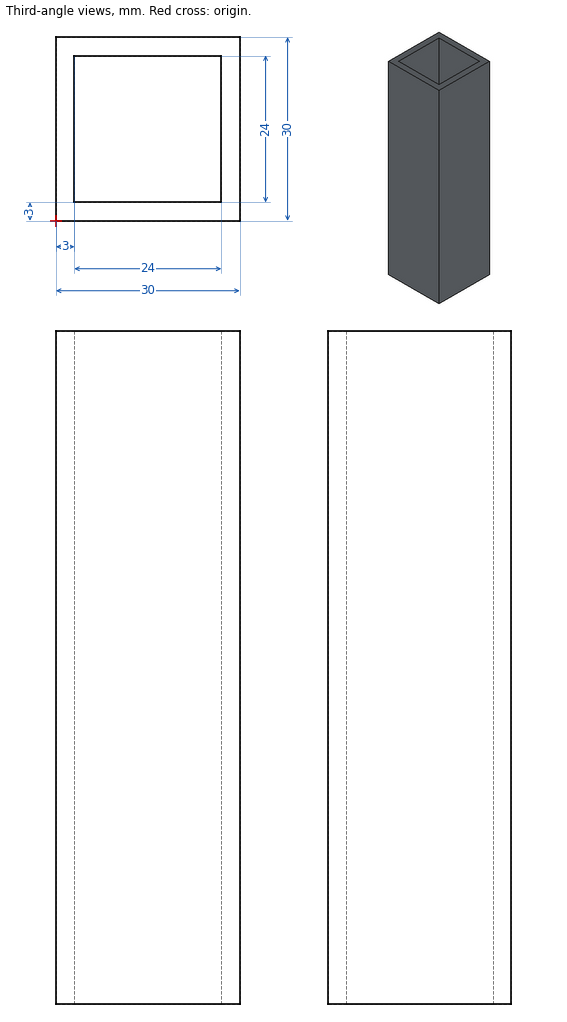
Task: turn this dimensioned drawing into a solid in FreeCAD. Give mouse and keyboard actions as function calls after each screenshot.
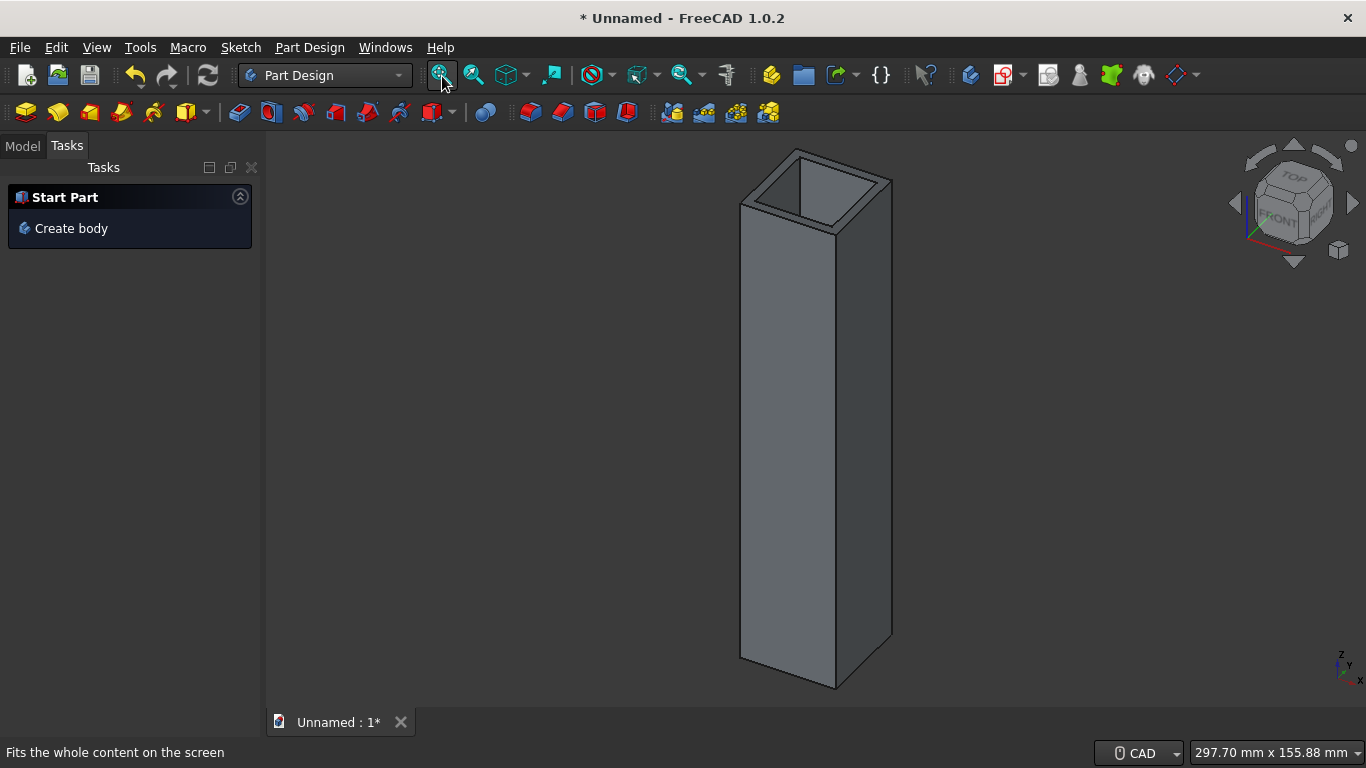
key(5)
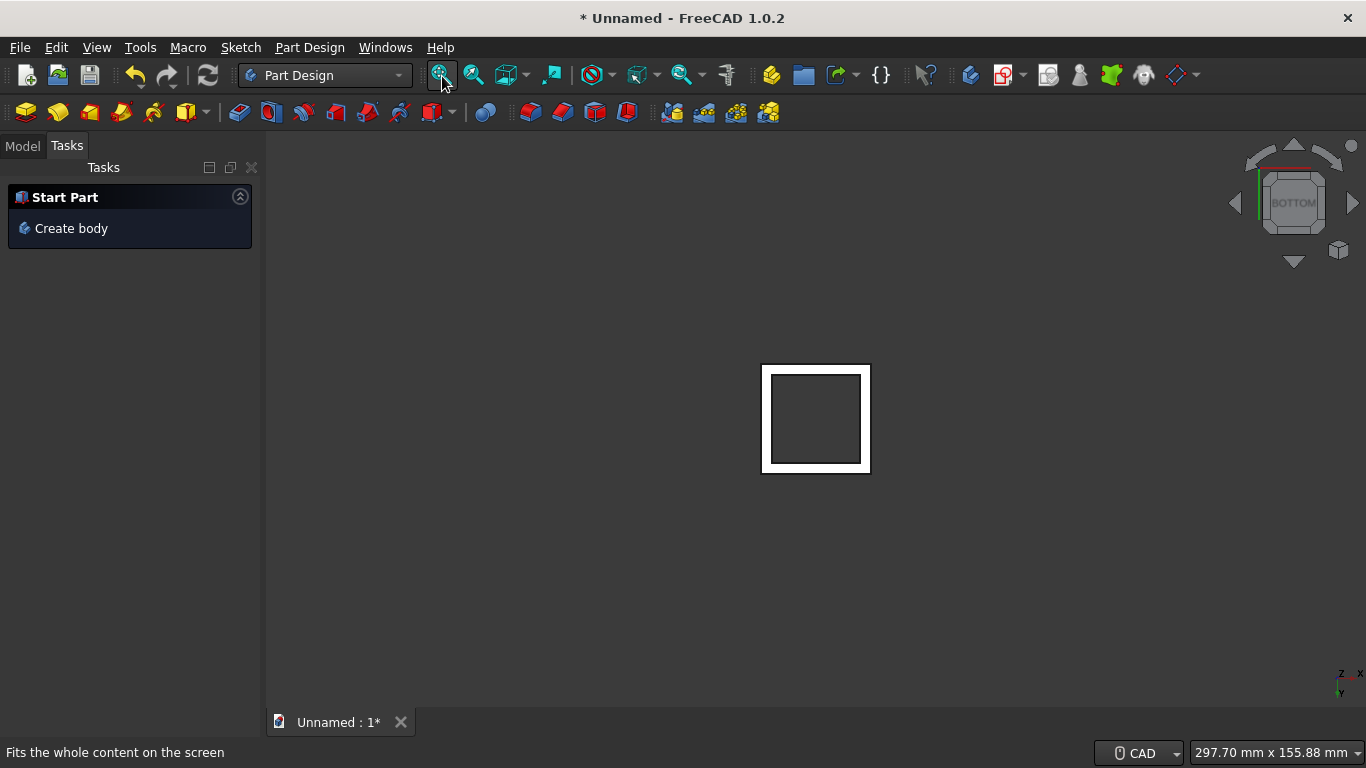
click(442, 76)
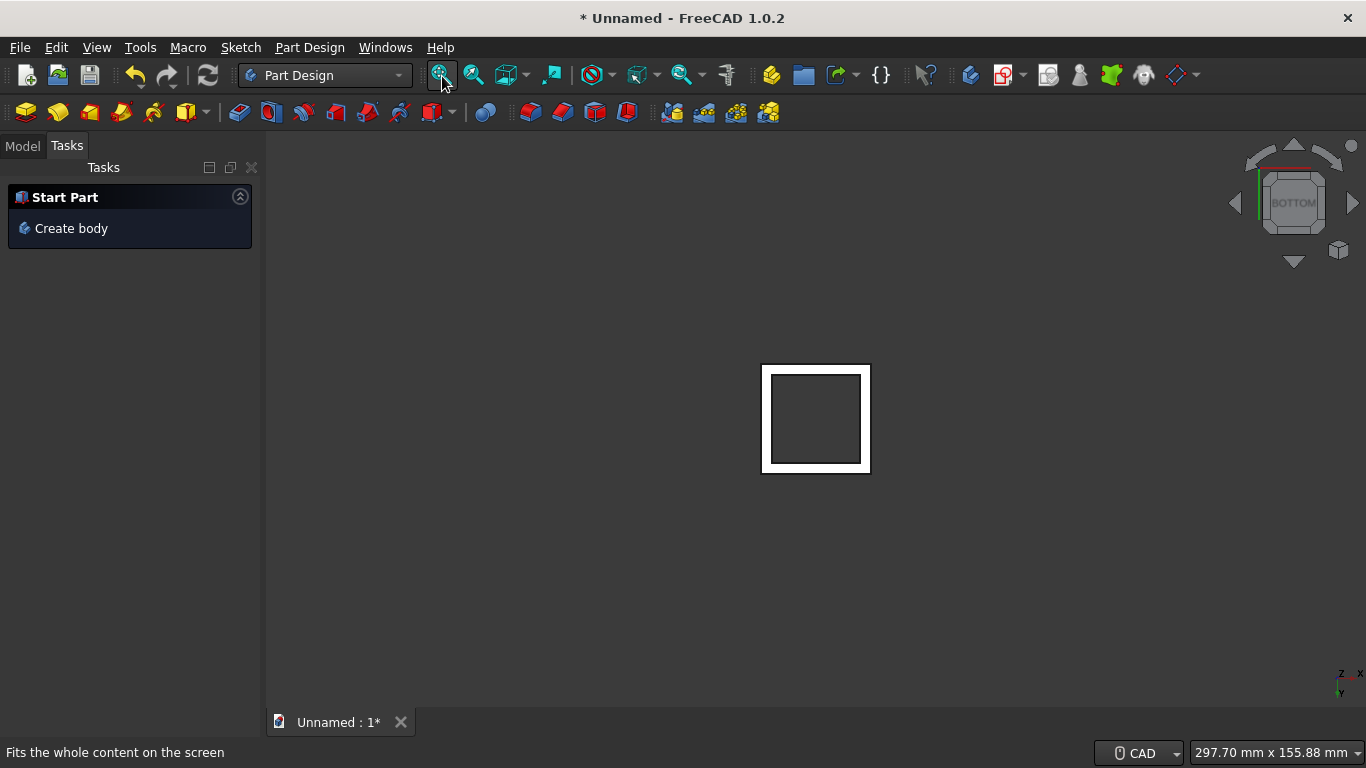
scroll(864, 466, up, 5)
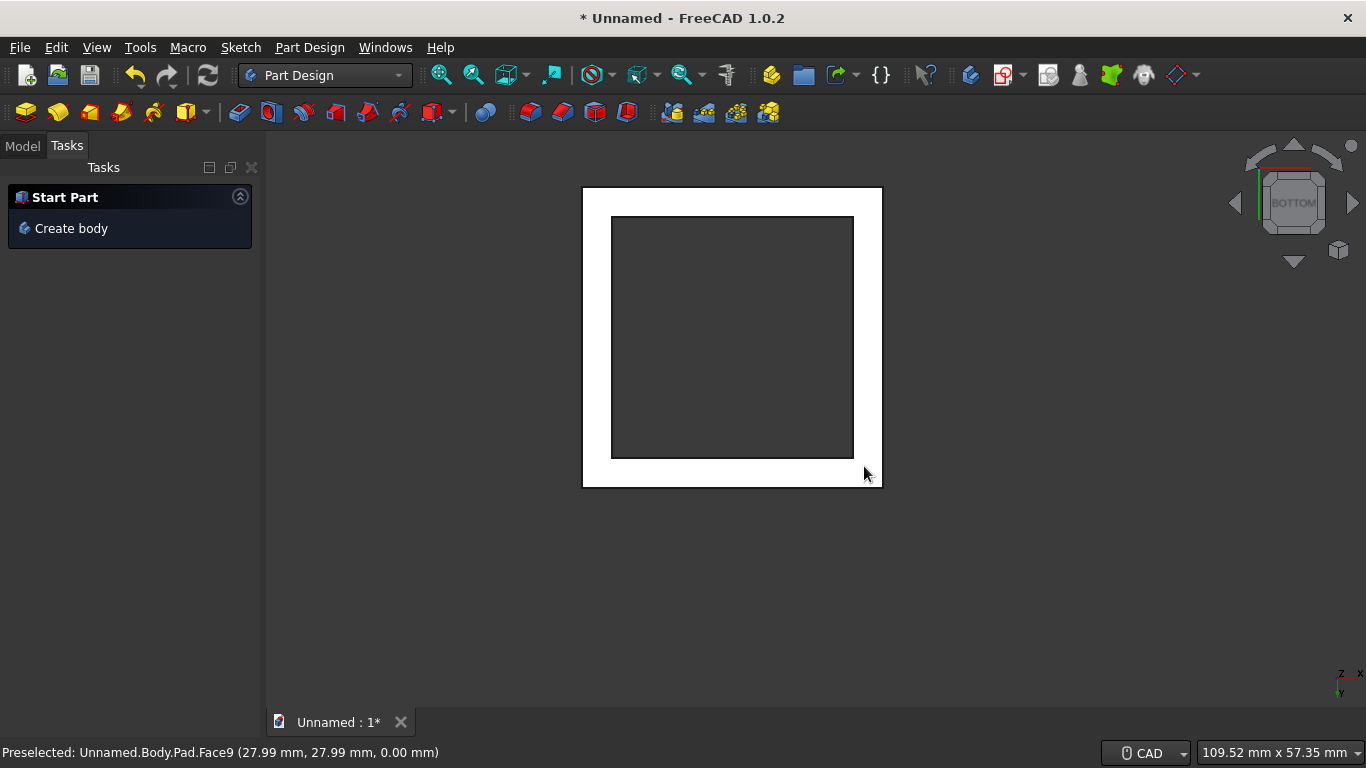
click(862, 465)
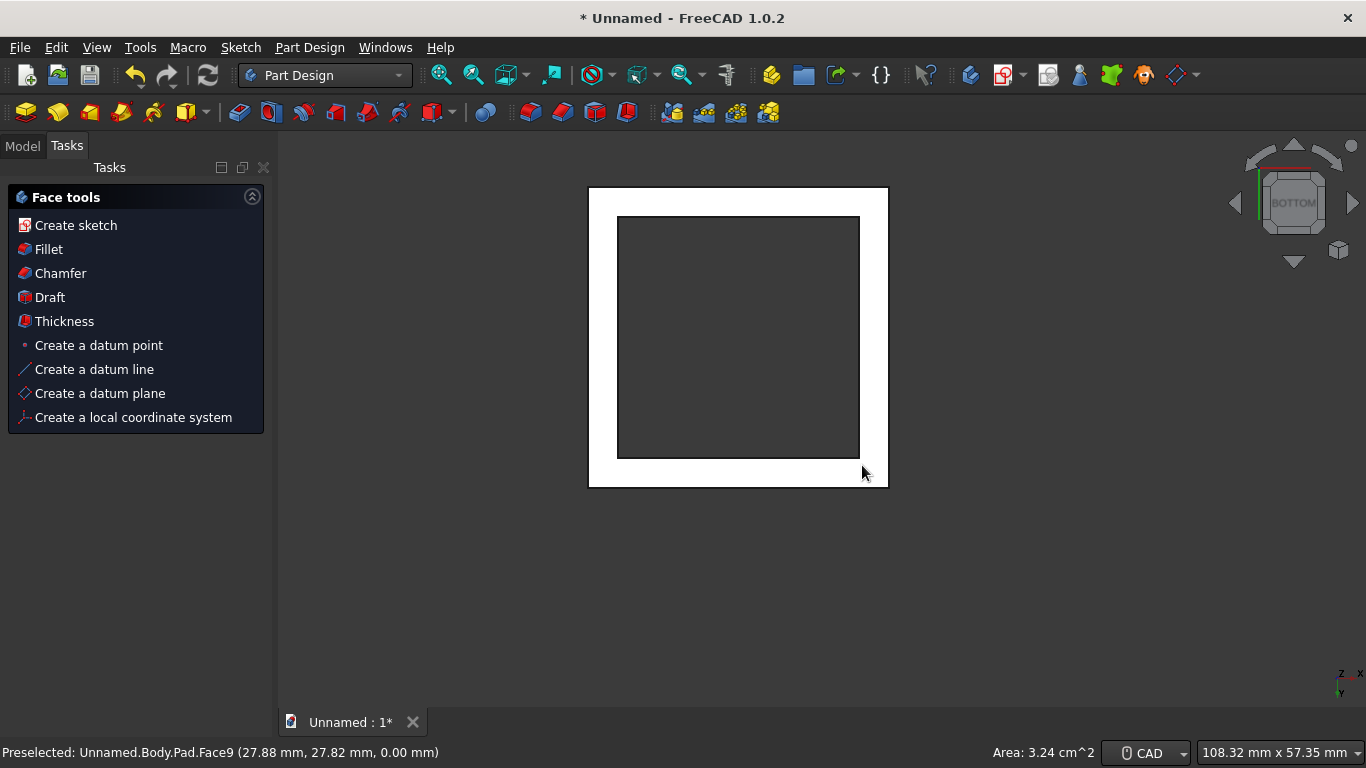
click(1004, 76)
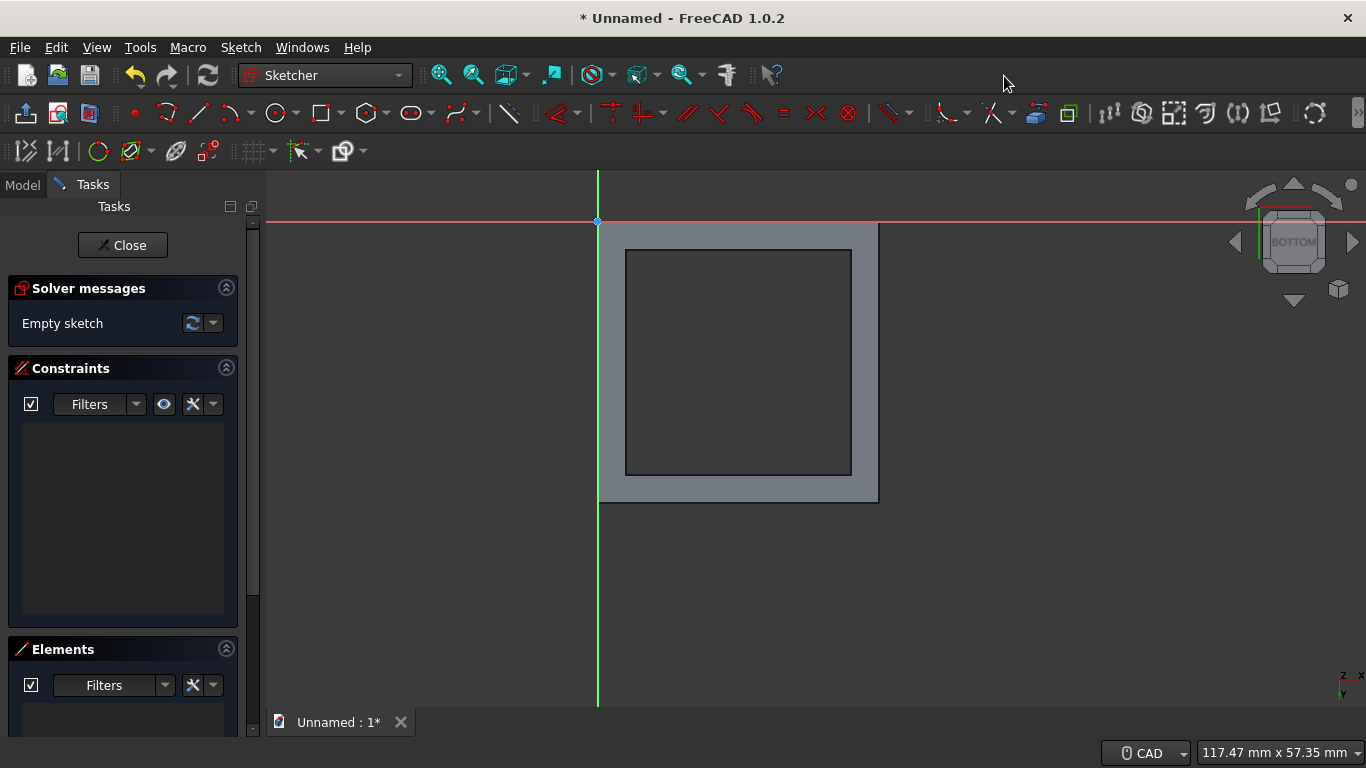
scroll(696, 198, up, 1)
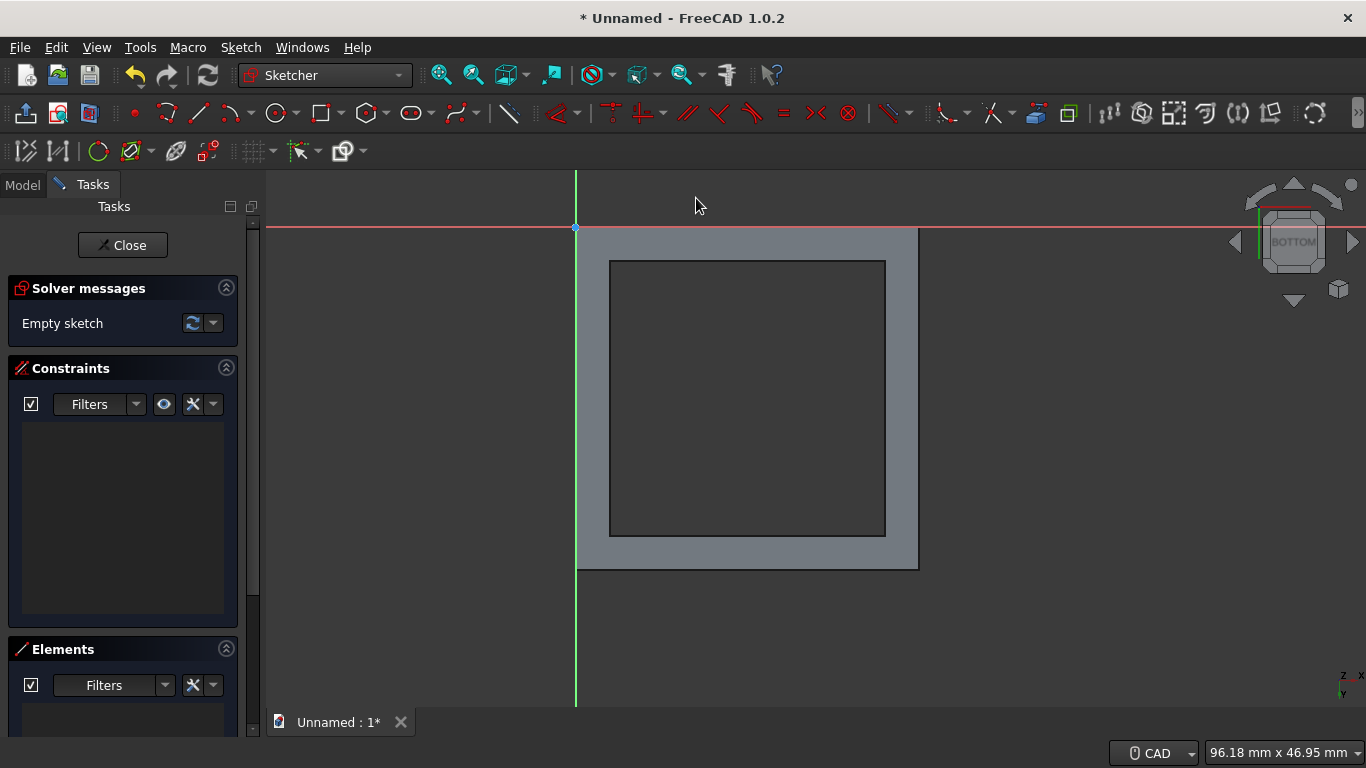
click(322, 114)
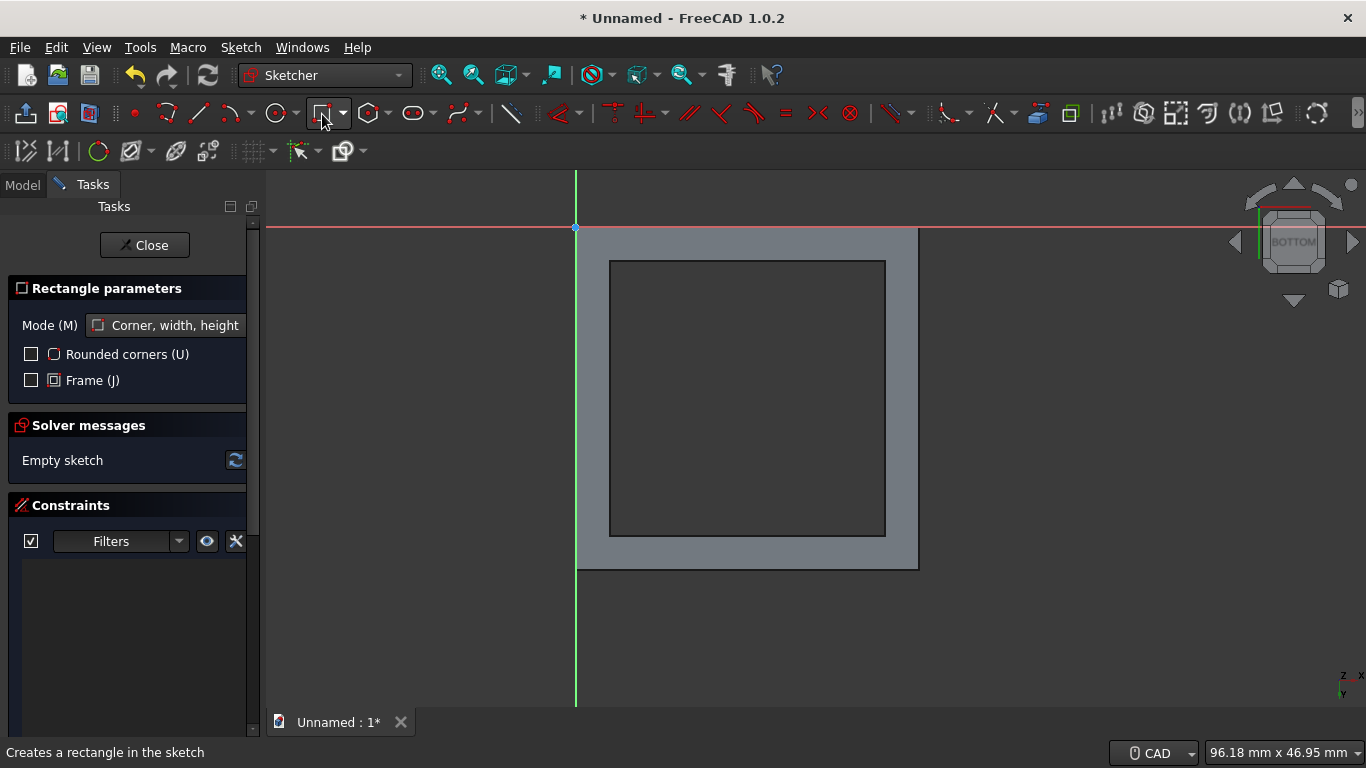
click(576, 227)
move(919, 570)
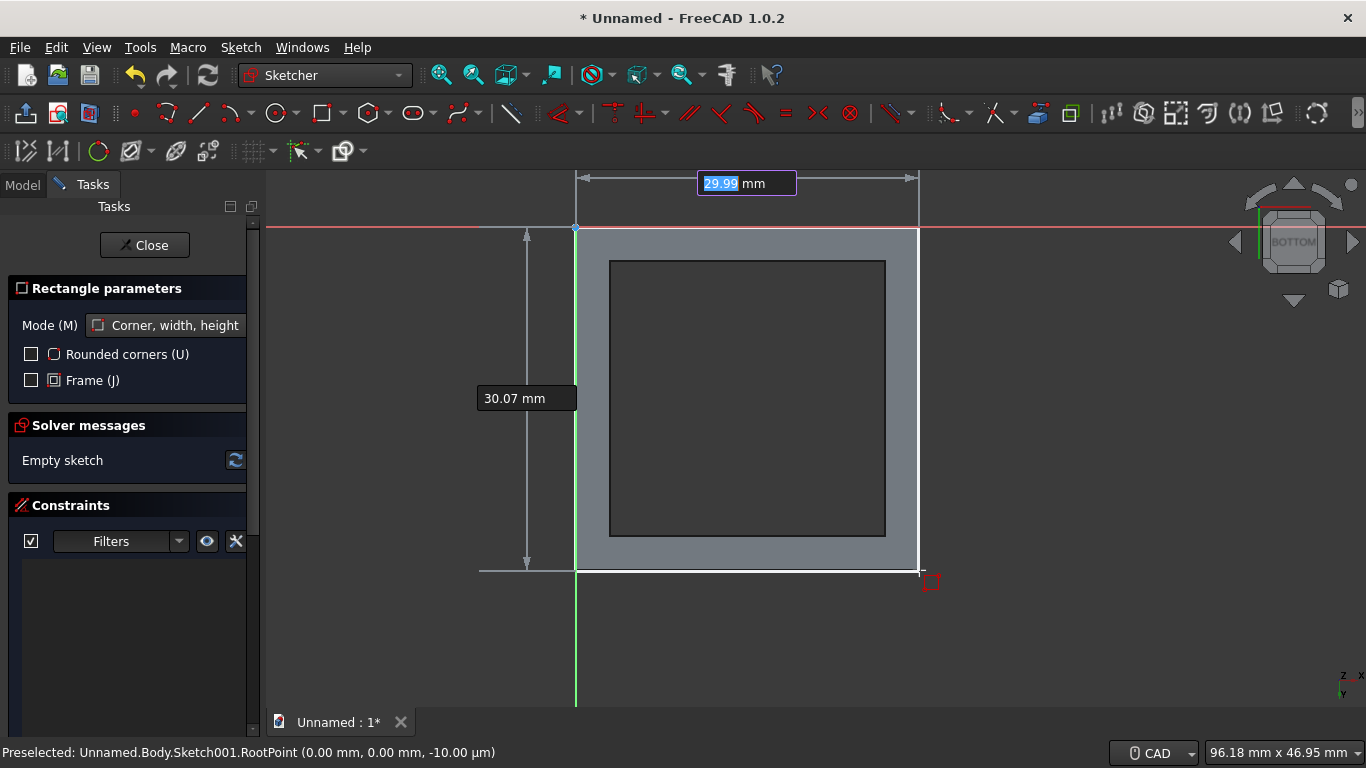
text(30)
key(Tab)
text(30)
key(Return)
key(Escape)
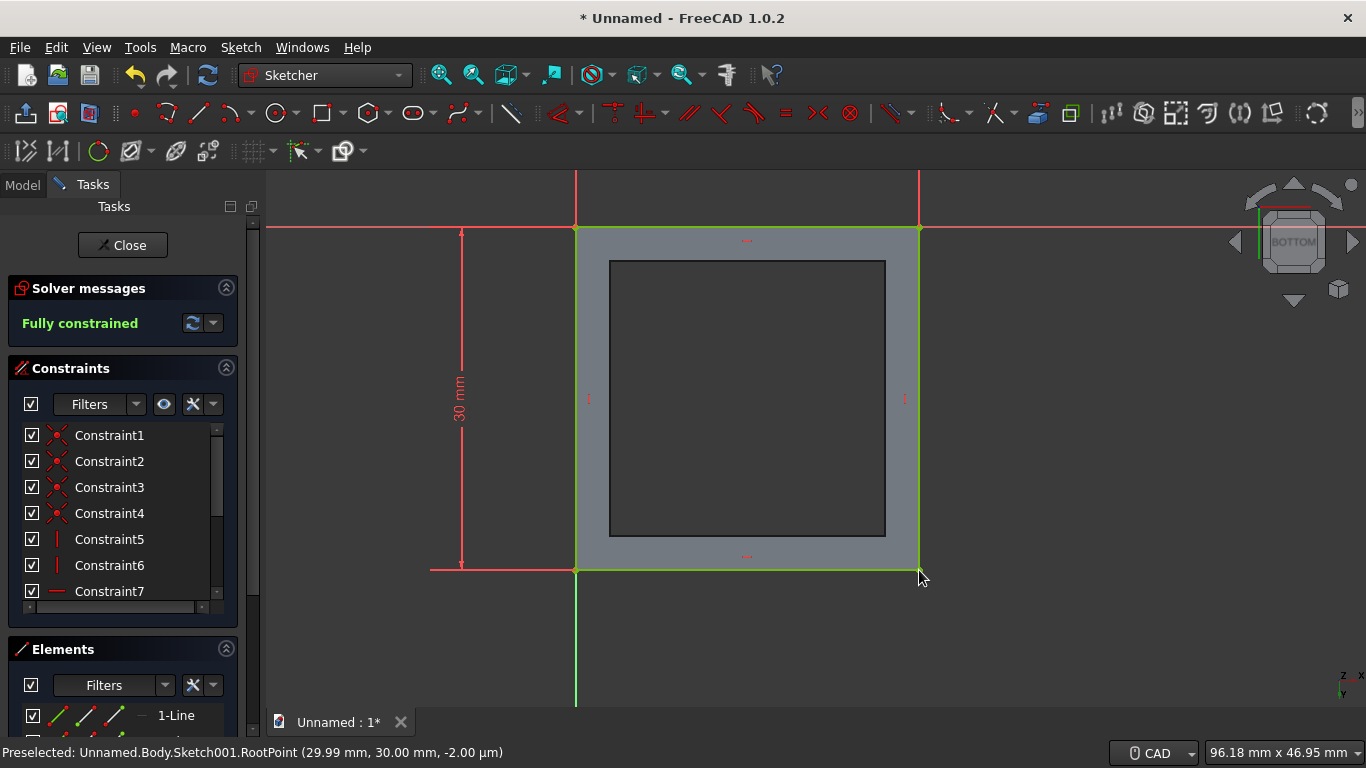
click(123, 245)